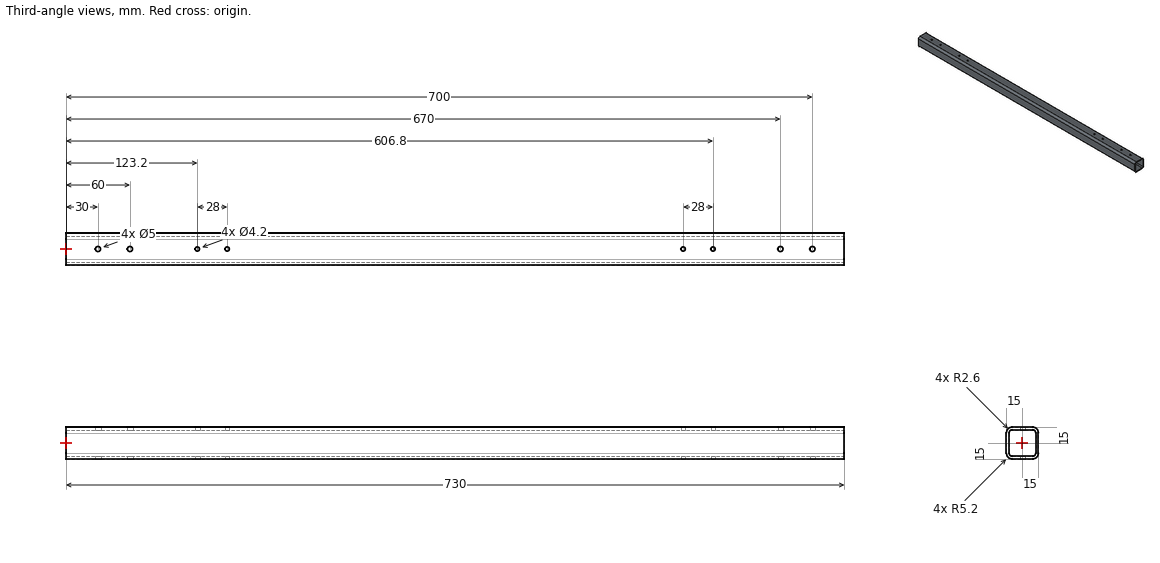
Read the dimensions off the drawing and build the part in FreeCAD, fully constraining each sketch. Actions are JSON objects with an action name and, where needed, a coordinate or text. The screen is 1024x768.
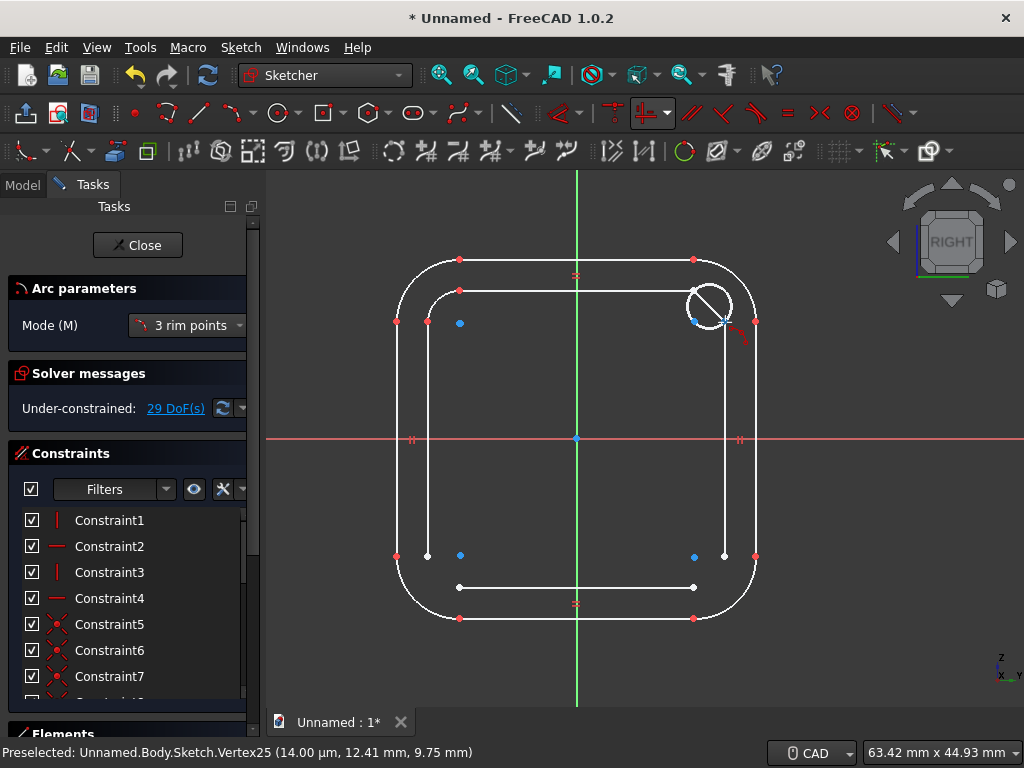
{"action": "scroll", "coordinate": [716, 299], "scroll_direction": "up", "scroll_amount": 3}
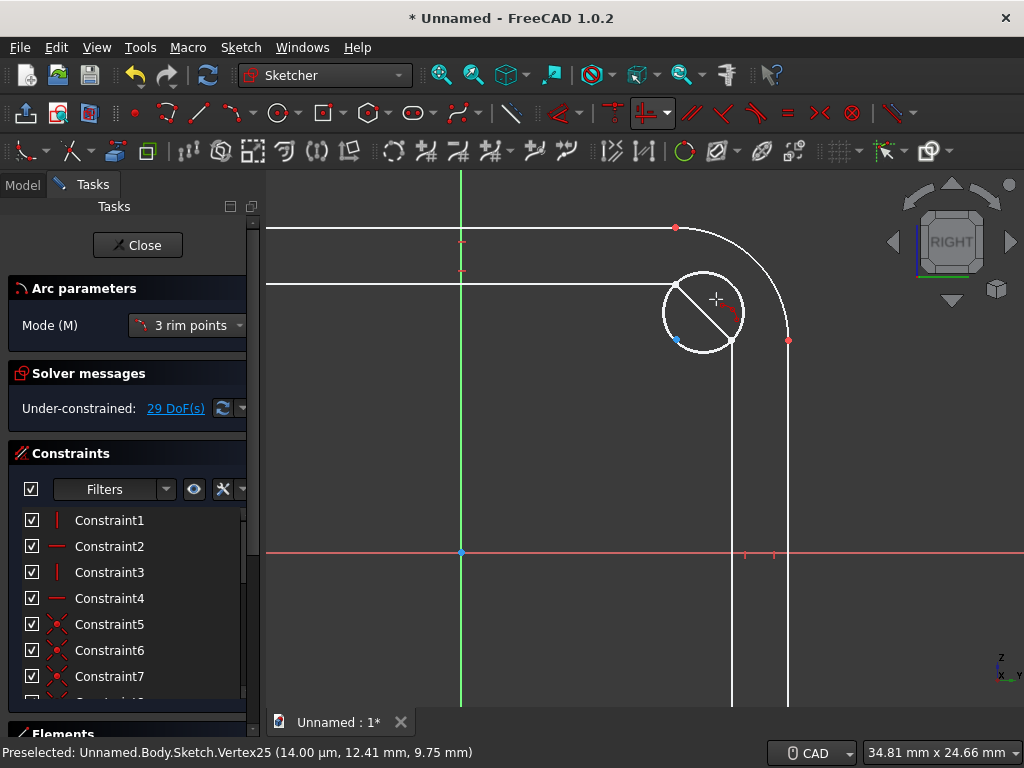
{"action": "left_click", "coordinate": [715, 300]}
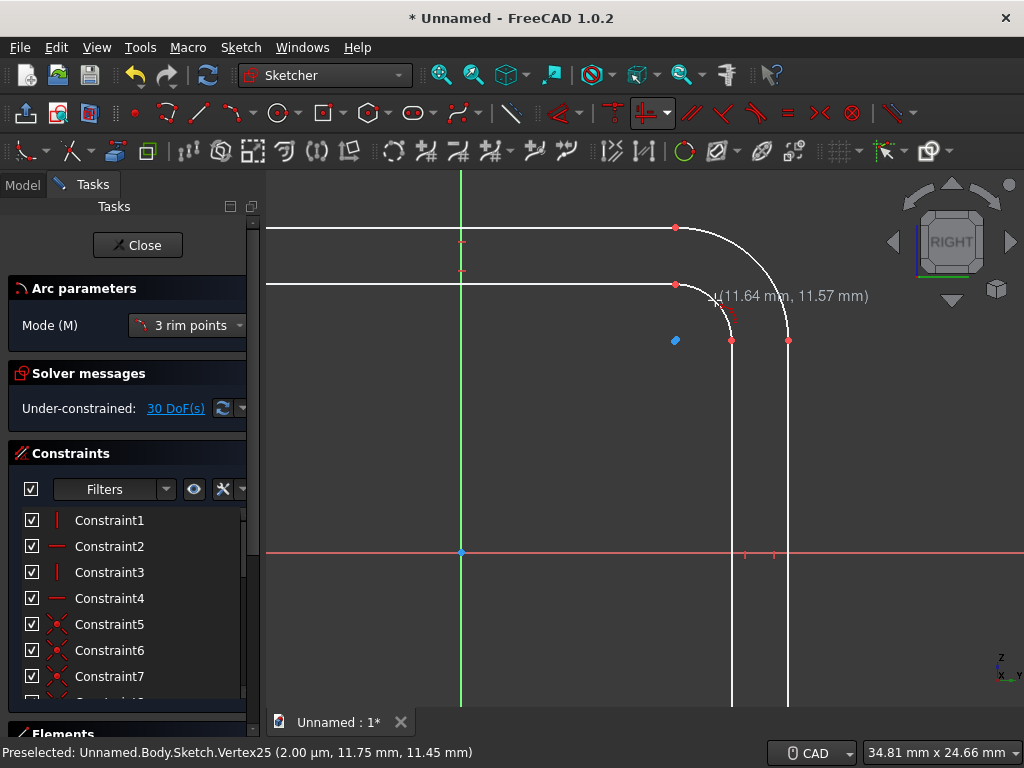
{"action": "scroll", "coordinate": [716, 299], "scroll_direction": "down", "scroll_amount": 3}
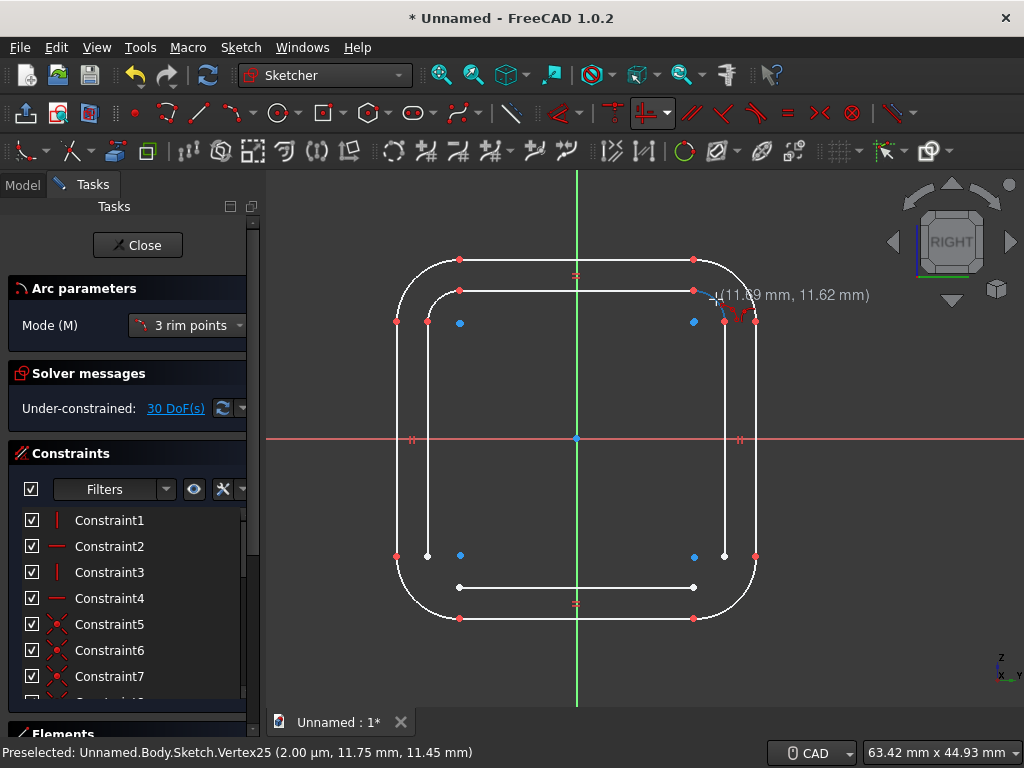
{"action": "left_click", "coordinate": [725, 557]}
{"action": "left_click", "coordinate": [694, 588]}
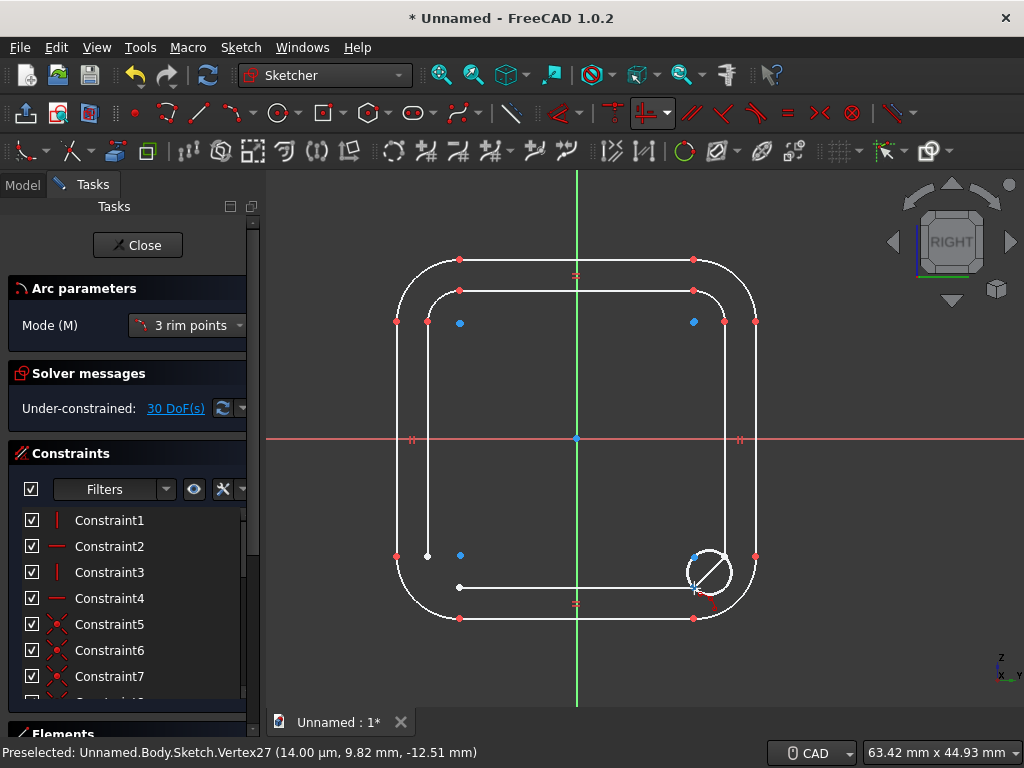
{"action": "scroll", "coordinate": [716, 578], "scroll_direction": "up", "scroll_amount": 3}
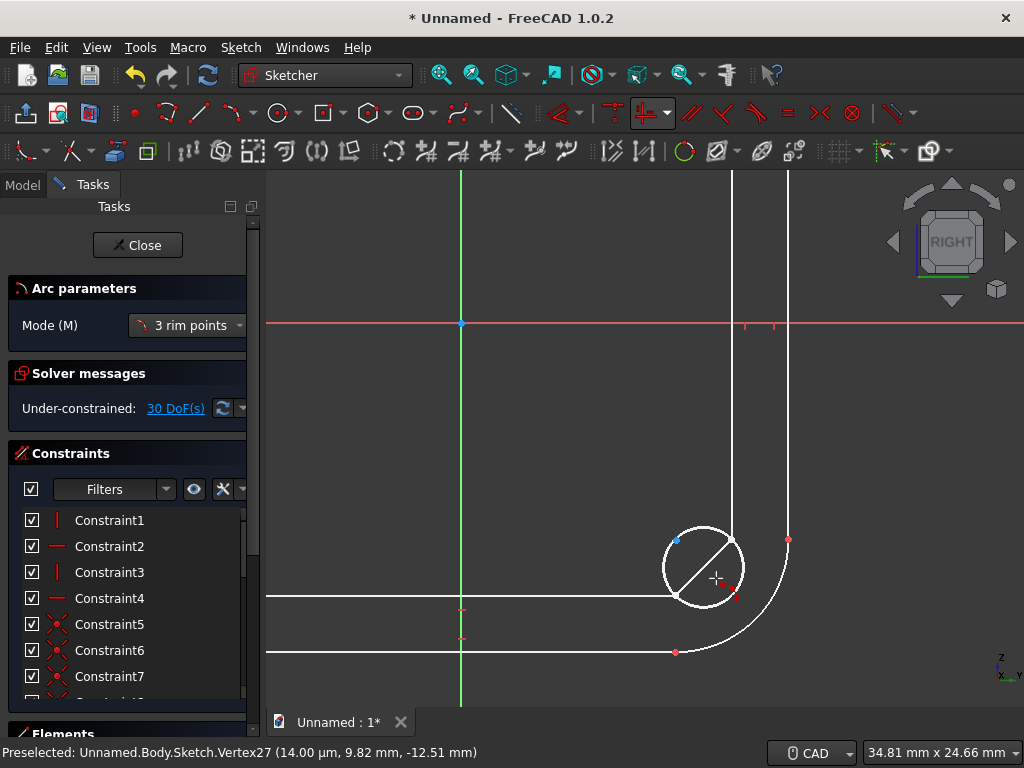
{"action": "left_click", "coordinate": [715, 577]}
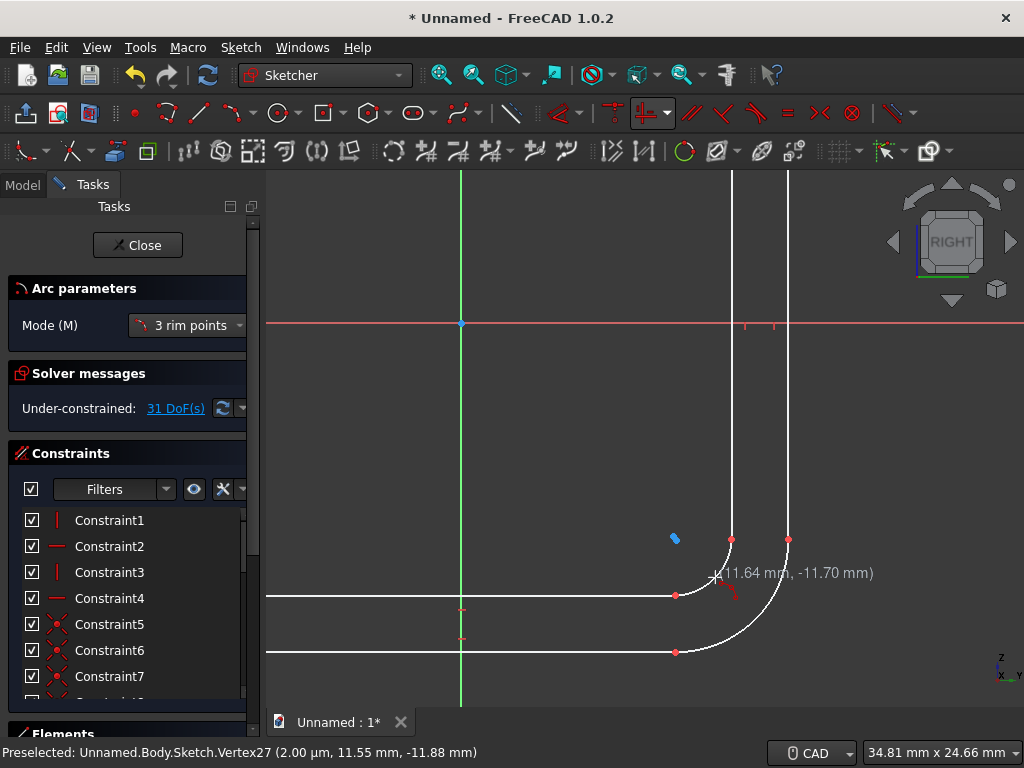
{"action": "scroll", "coordinate": [716, 579], "scroll_direction": "down", "scroll_amount": 3}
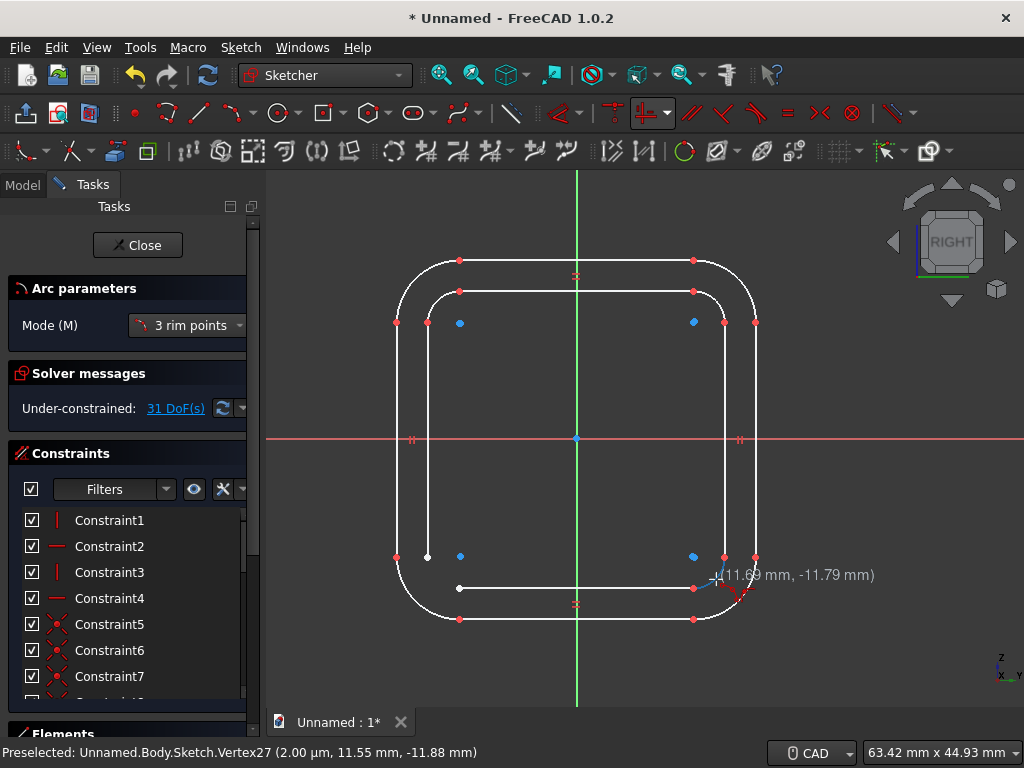
{"action": "left_click", "coordinate": [460, 588]}
{"action": "left_click", "coordinate": [428, 557]}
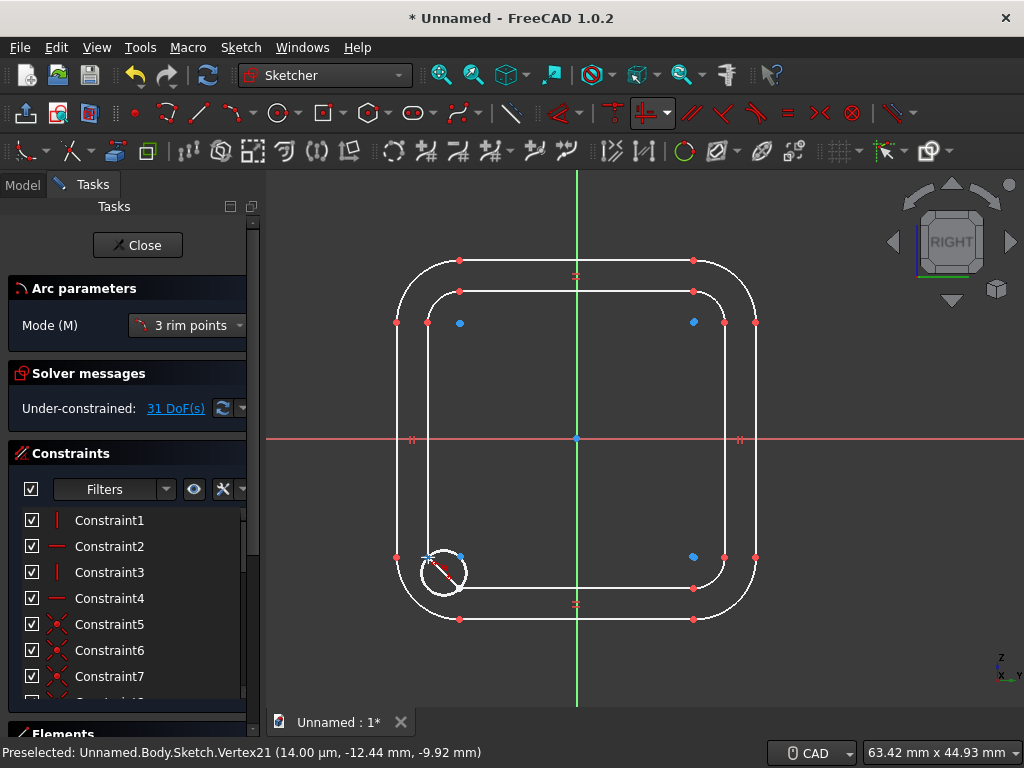
{"action": "scroll", "coordinate": [437, 578], "scroll_direction": "up", "scroll_amount": 3}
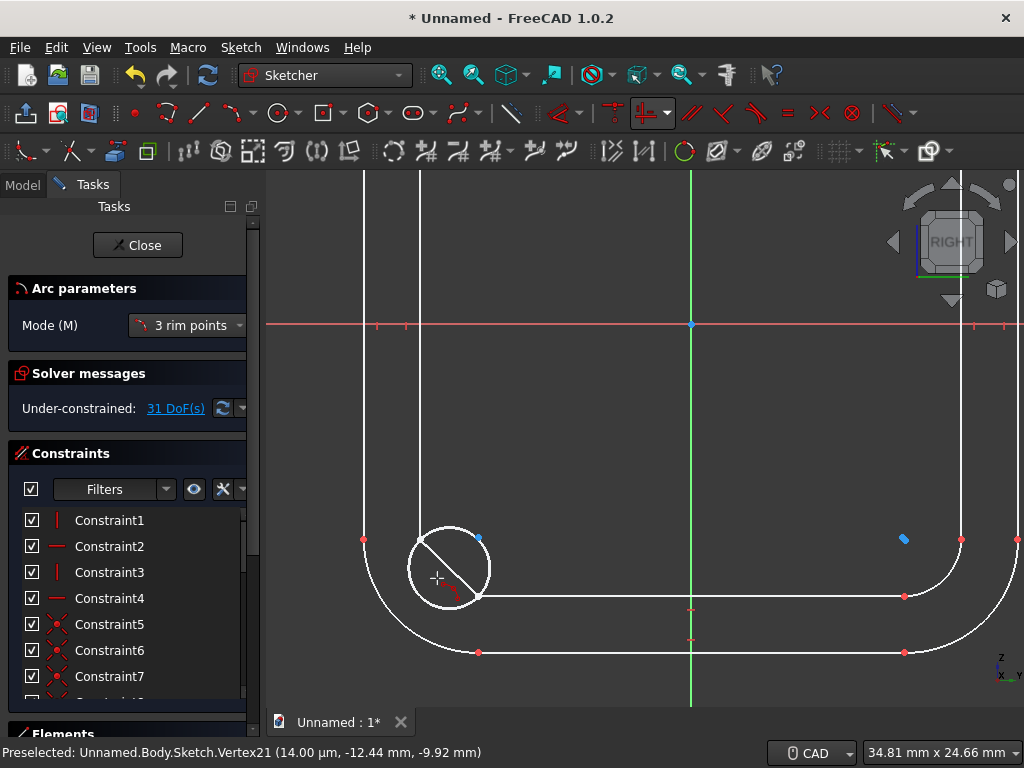
{"action": "left_click", "coordinate": [438, 577]}
{"action": "key", "text": "Escape"}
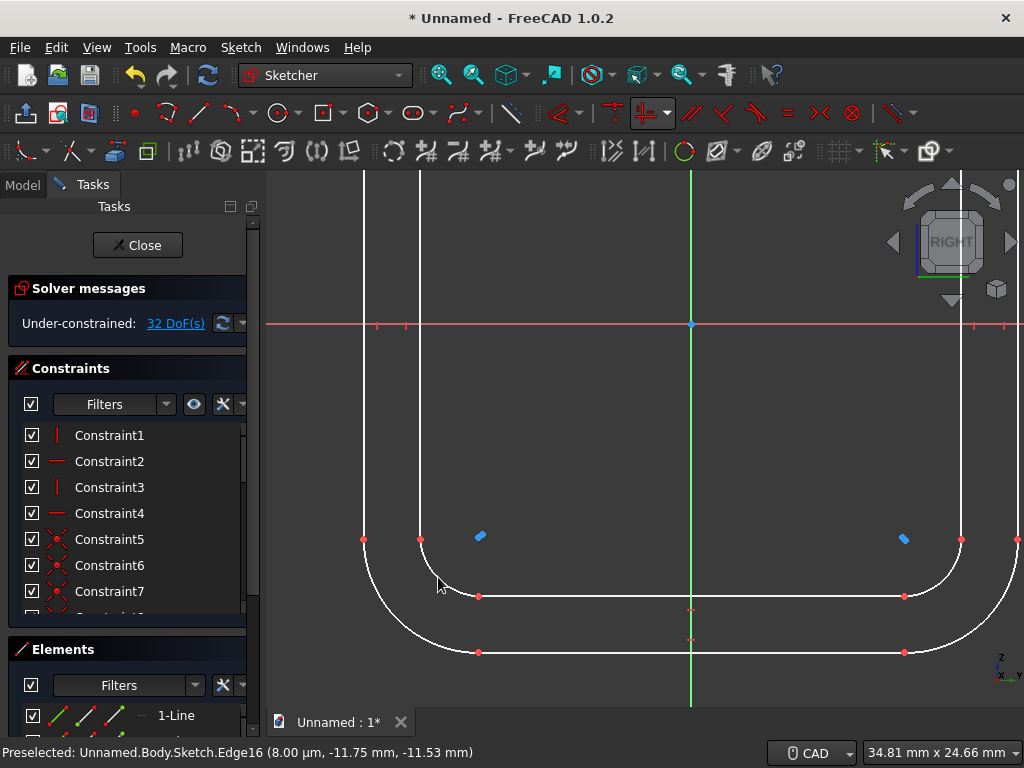
{"action": "left_click", "coordinate": [364, 240]}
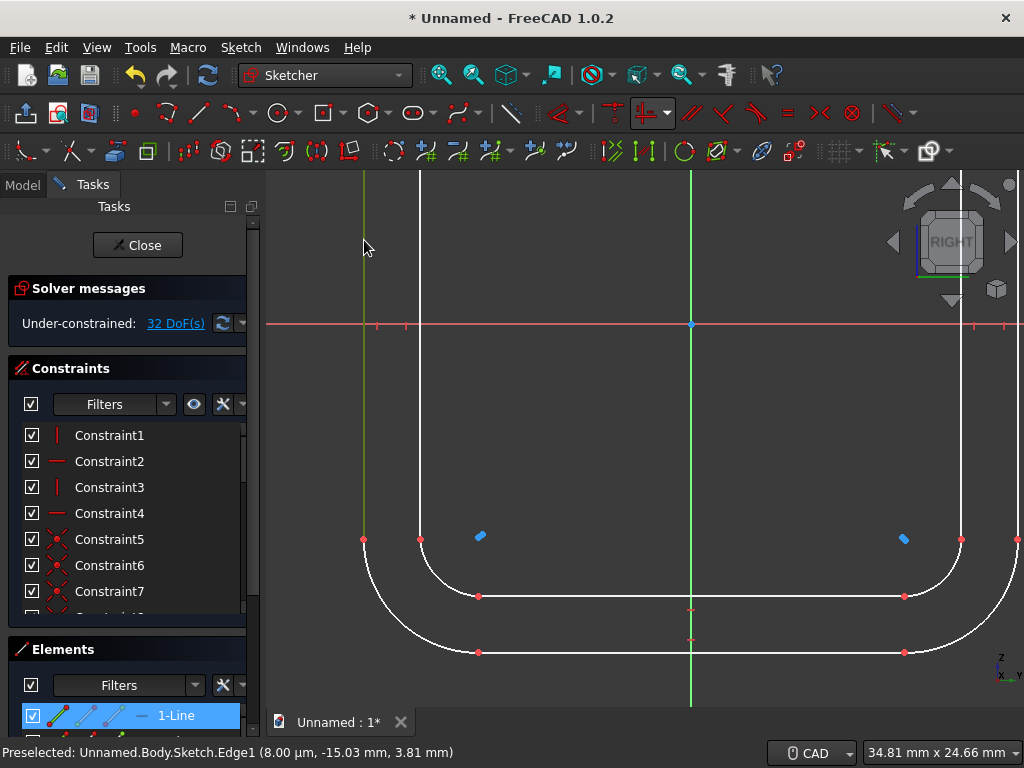
{"action": "left_click", "coordinate": [377, 591]}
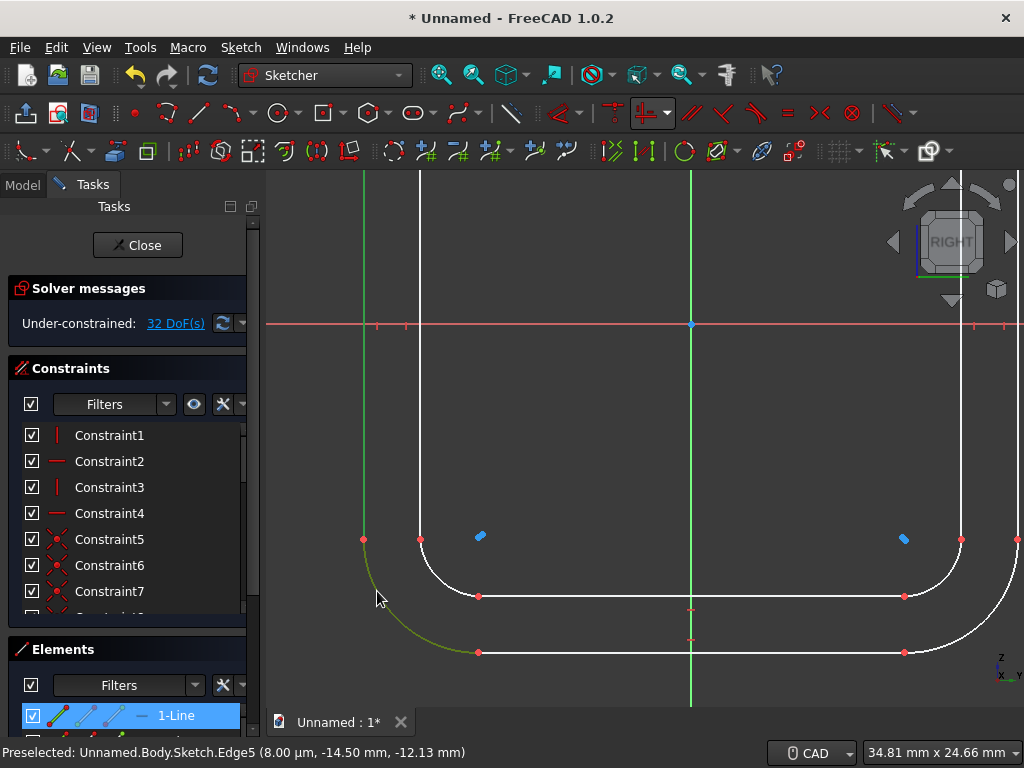
{"action": "left_click", "coordinate": [756, 114]}